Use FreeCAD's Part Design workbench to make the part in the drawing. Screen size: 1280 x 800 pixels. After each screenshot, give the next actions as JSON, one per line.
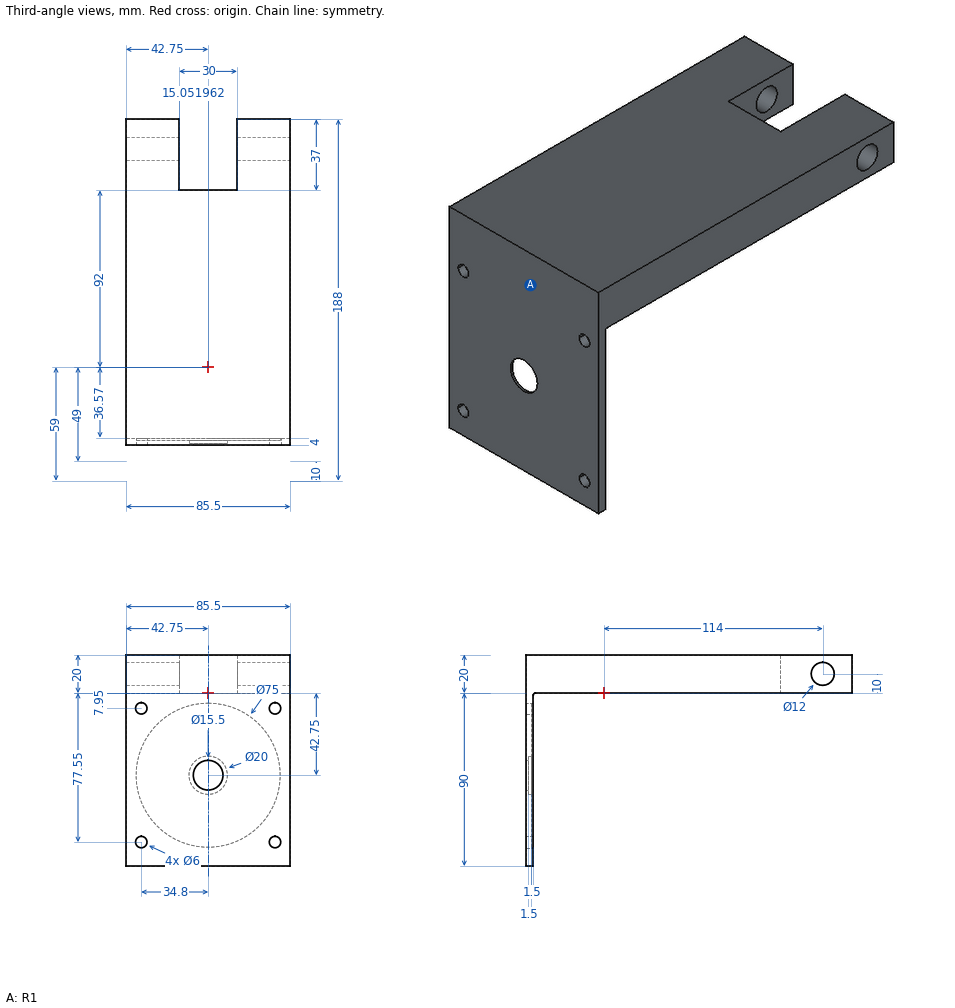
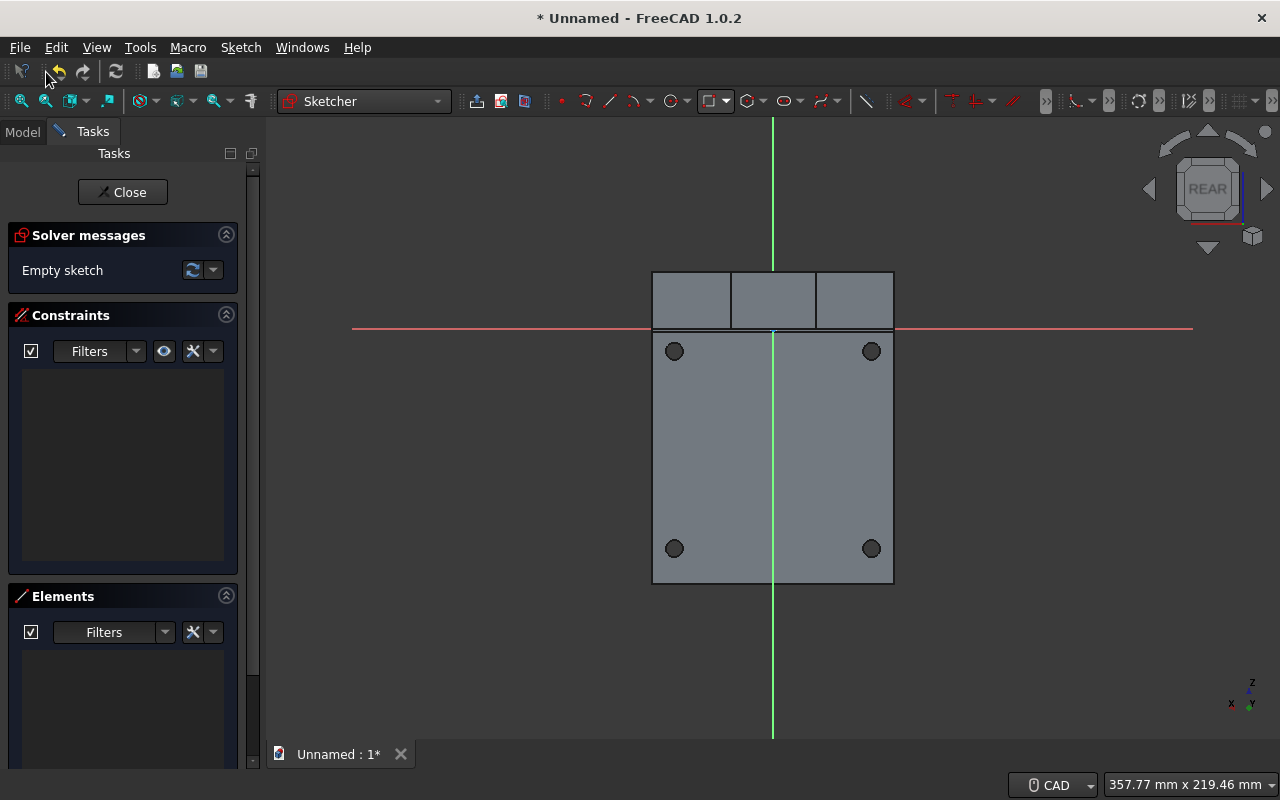
{"action": "scroll", "coordinate": [856, 460], "scroll_direction": "up", "scroll_amount": 3}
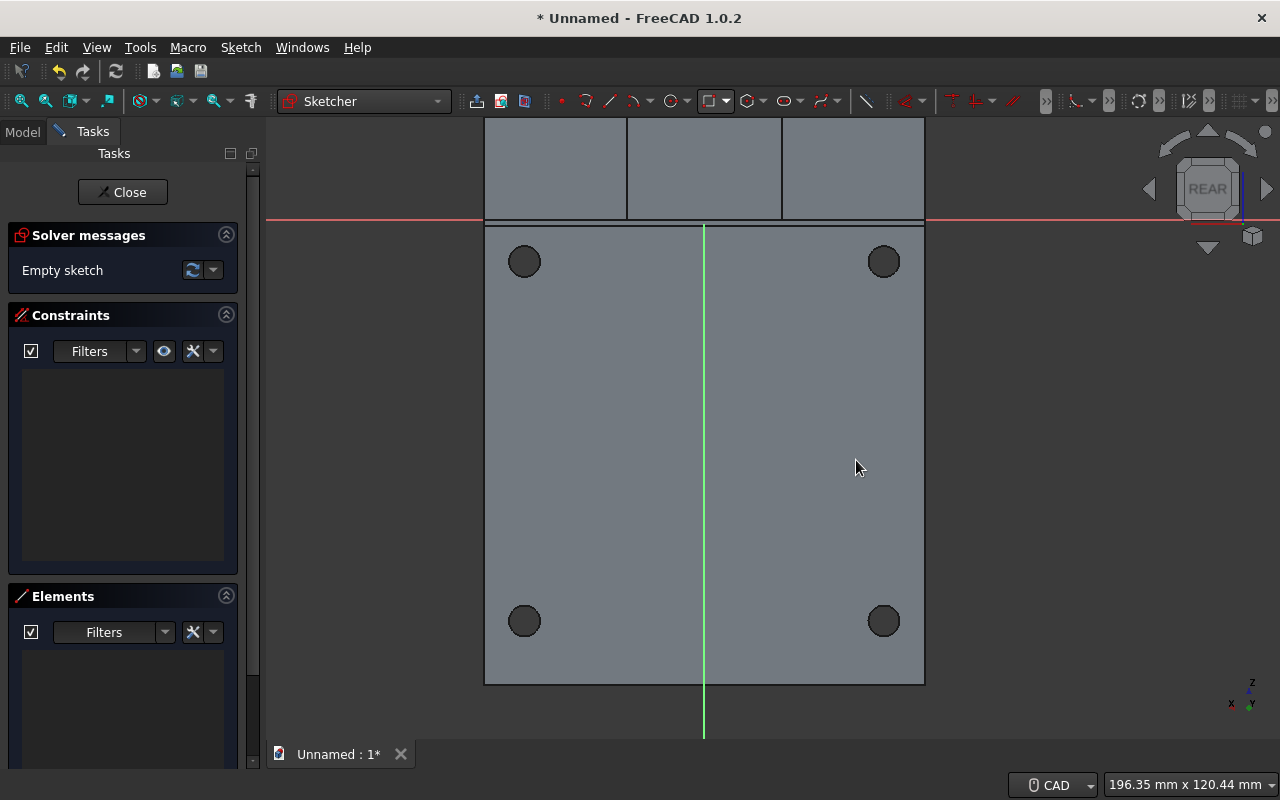
{"action": "key", "text": "g c"}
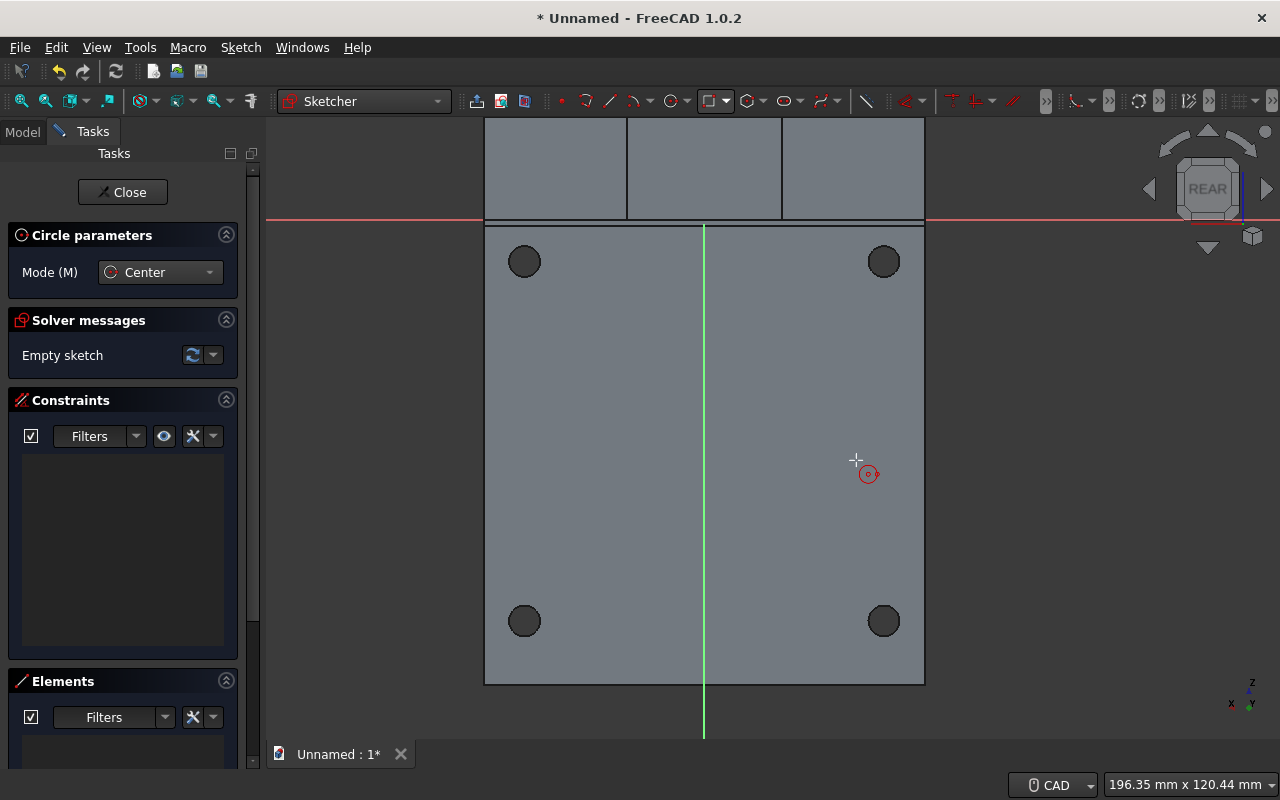
{"action": "left_click", "coordinate": [704, 441]}
{"action": "mouse_move", "coordinate": [841, 304]}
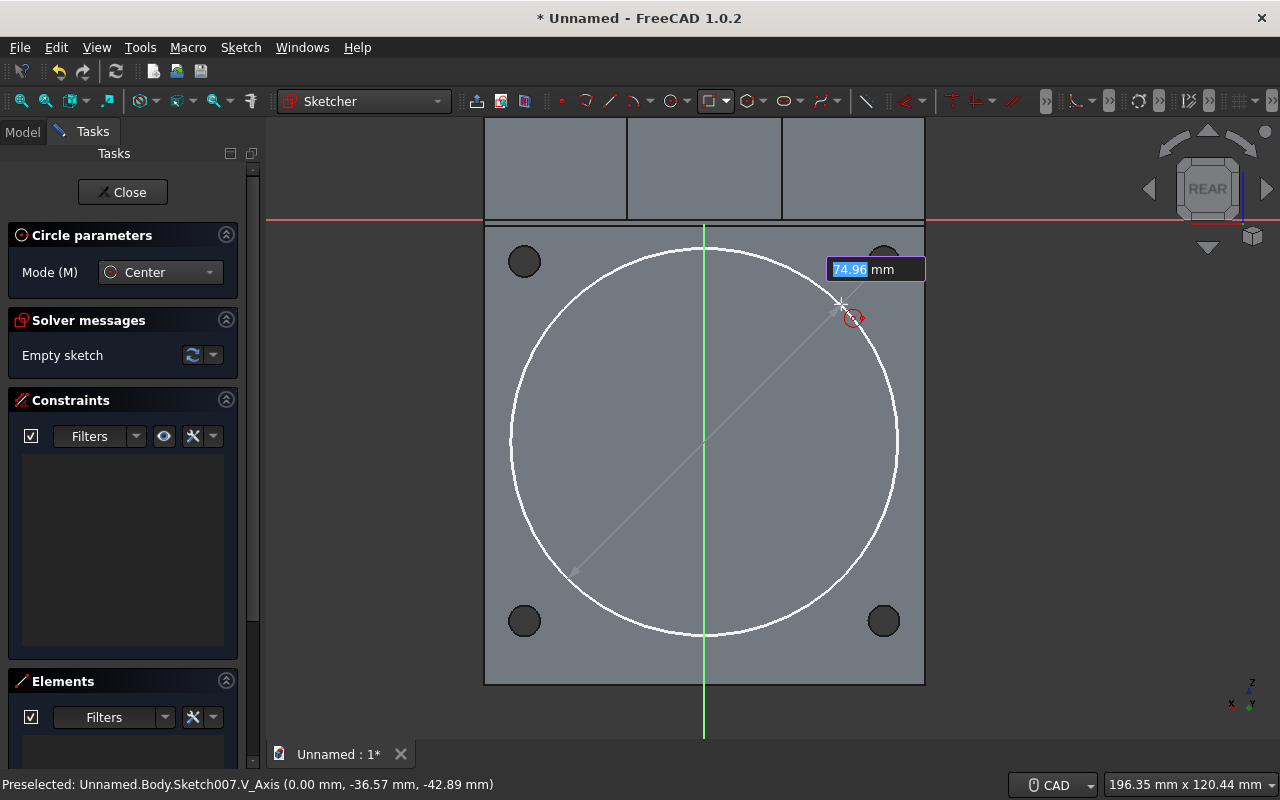
{"action": "type", "text": "75"}
{"action": "key", "text": "Return"}
{"action": "key", "text": "Escape"}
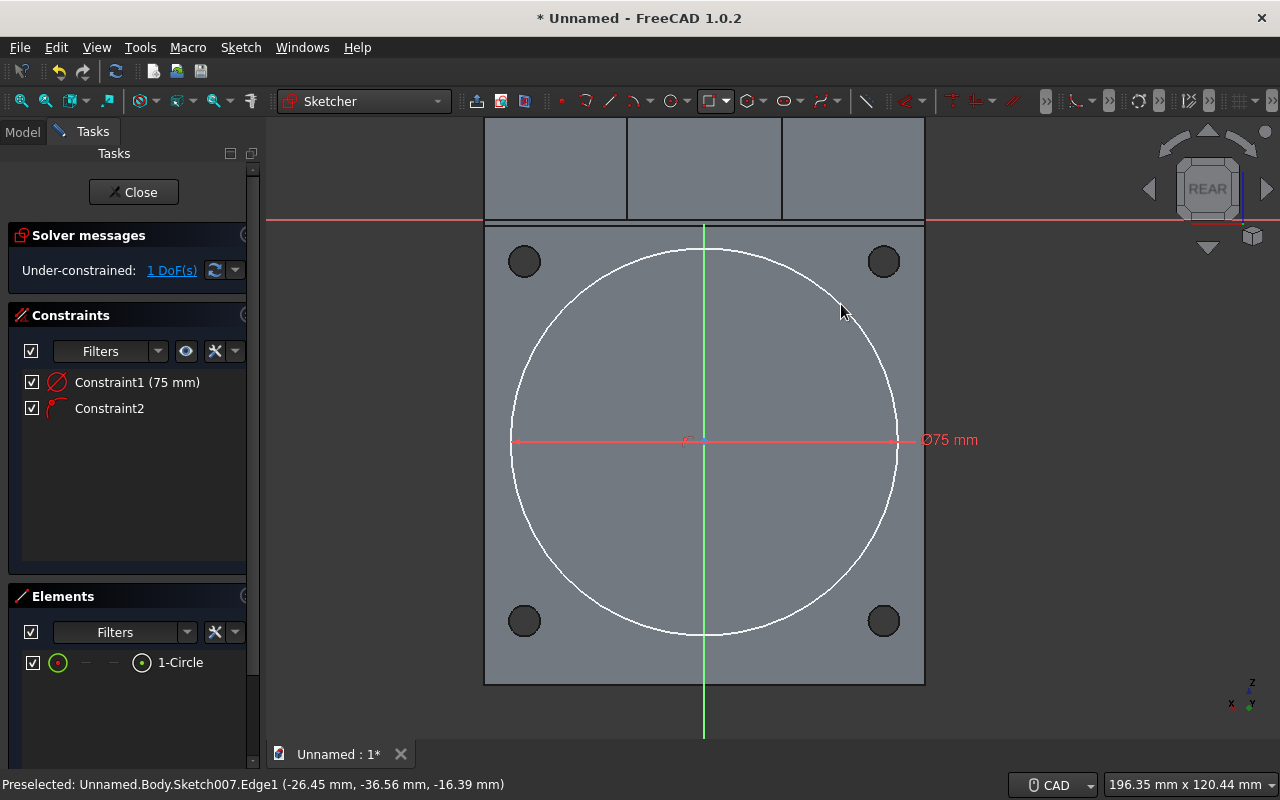
{"action": "key", "text": "d"}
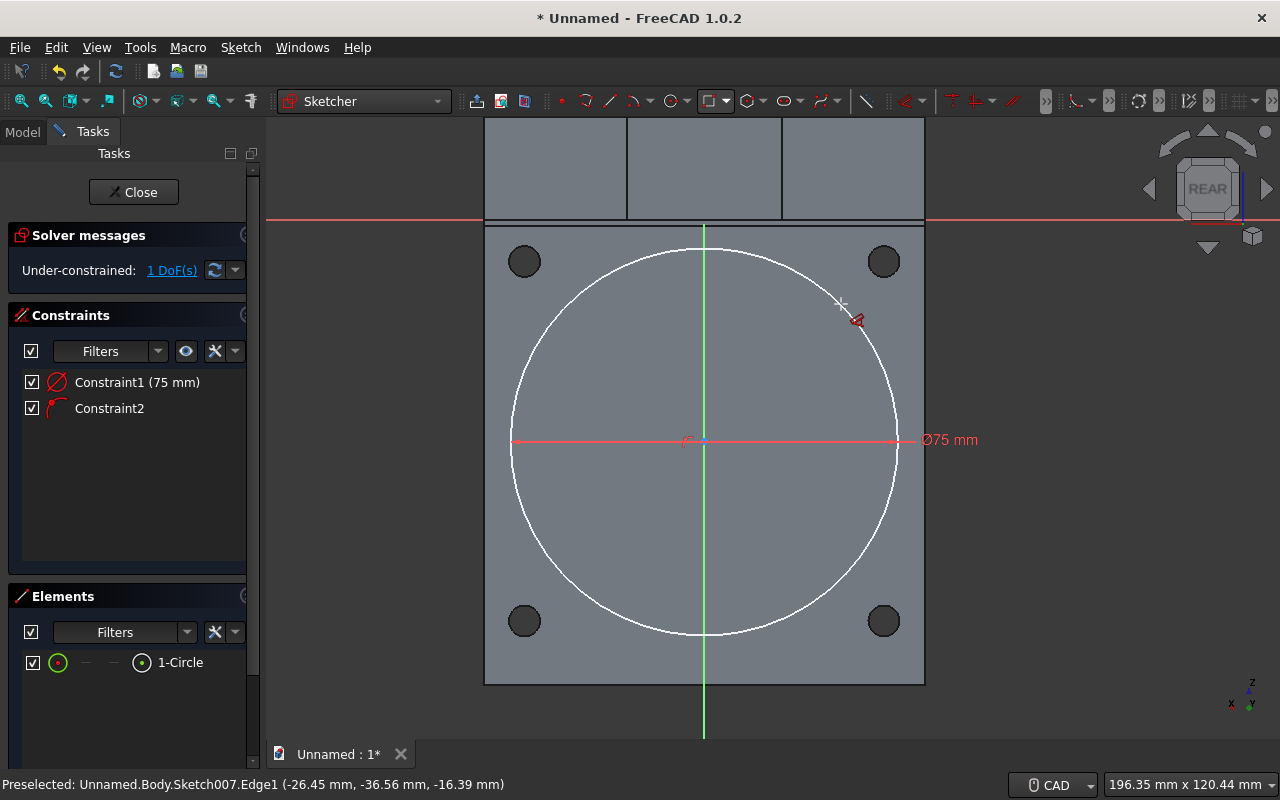
{"action": "left_click", "coordinate": [704, 442]}
{"action": "left_click", "coordinate": [738, 331]}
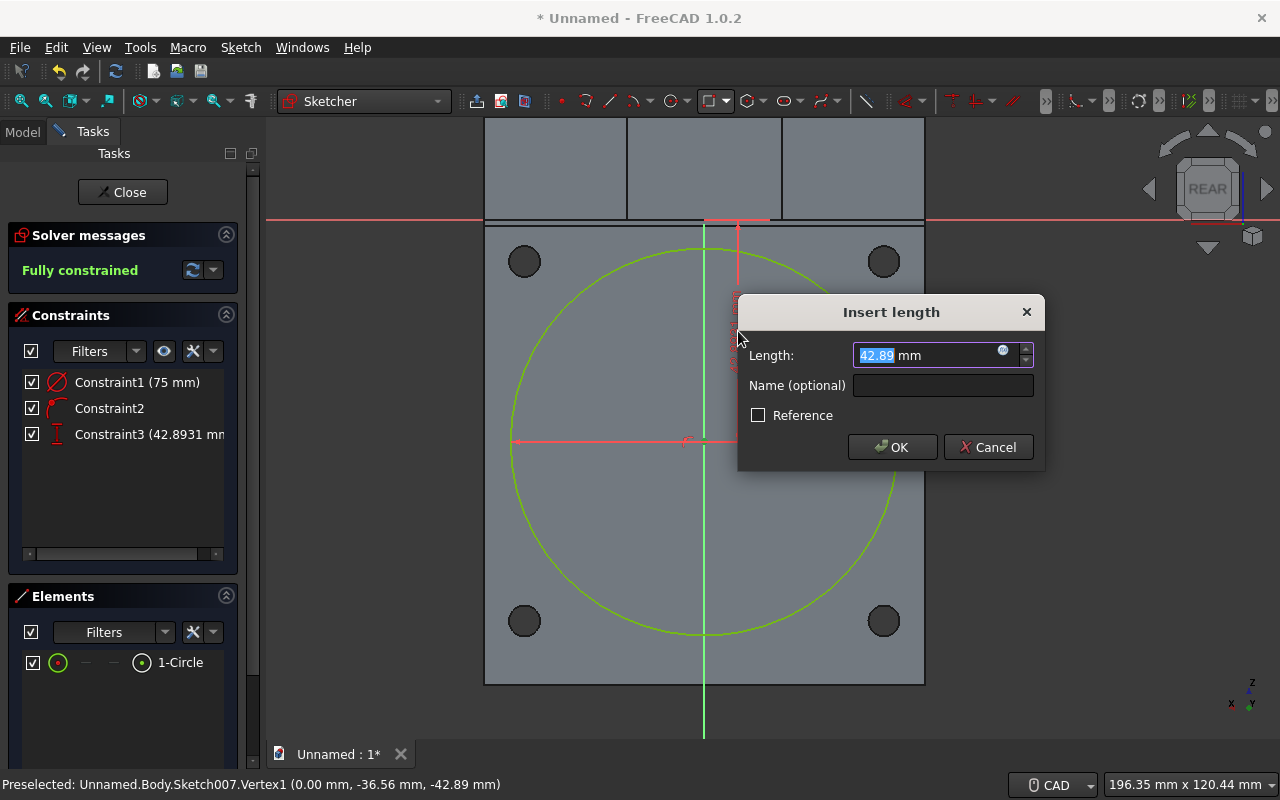
{"action": "type", "text": "42.75"}
{"action": "key", "text": "Return"}
{"action": "key", "text": "Escape"}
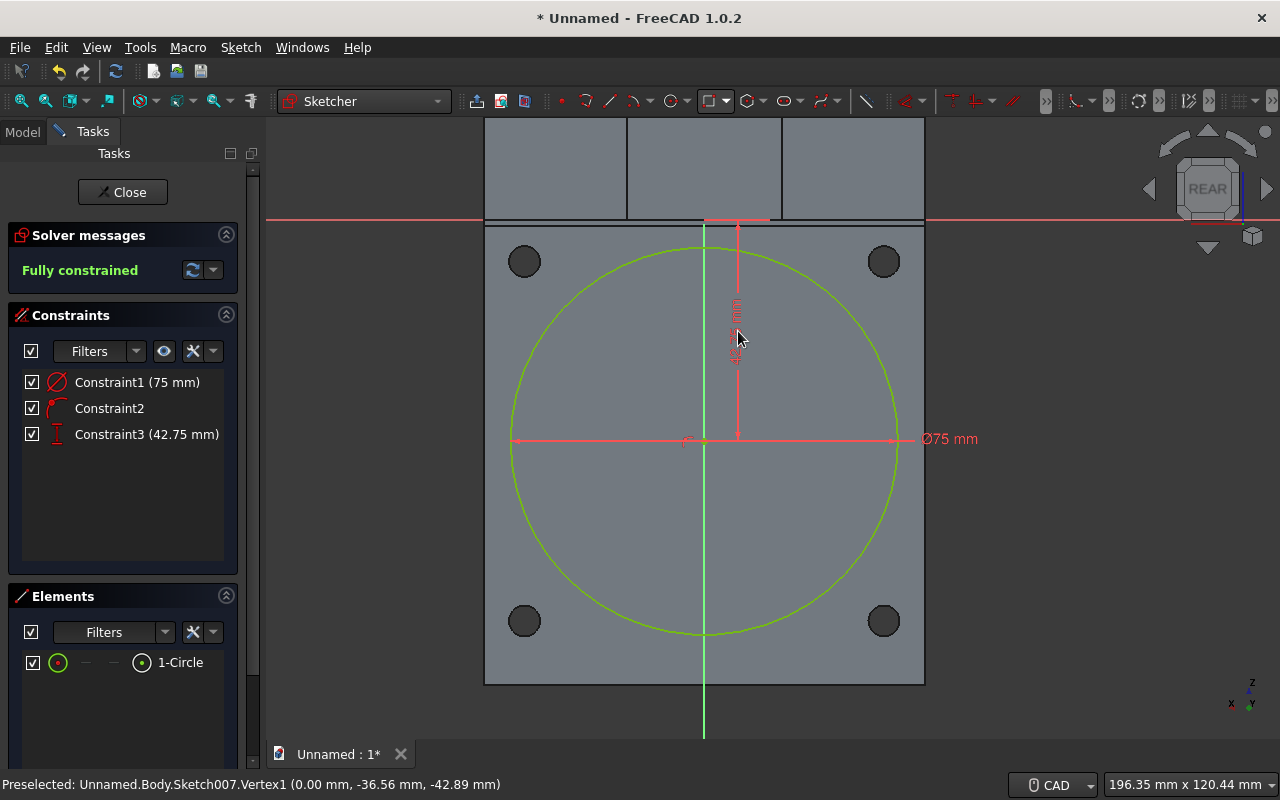
{"action": "left_click", "coordinate": [123, 192]}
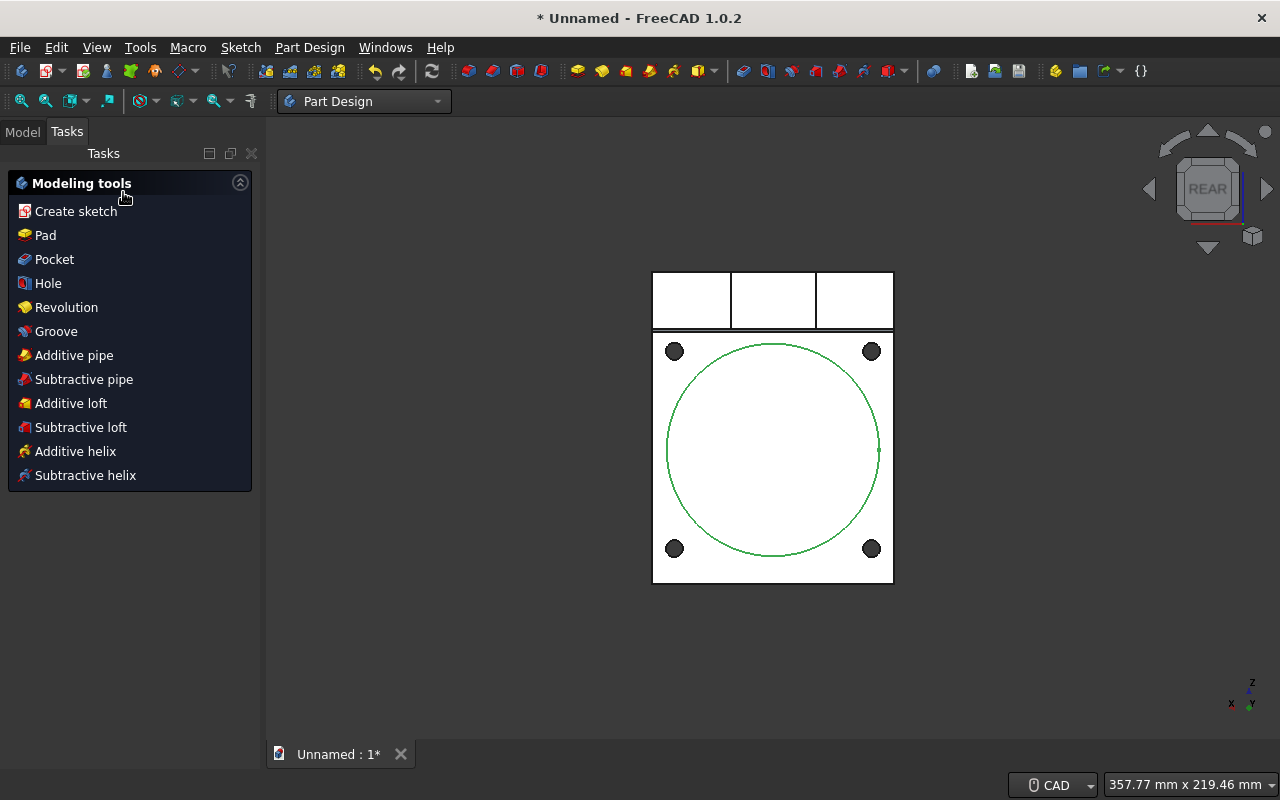
{"action": "left_click", "coordinate": [744, 72]}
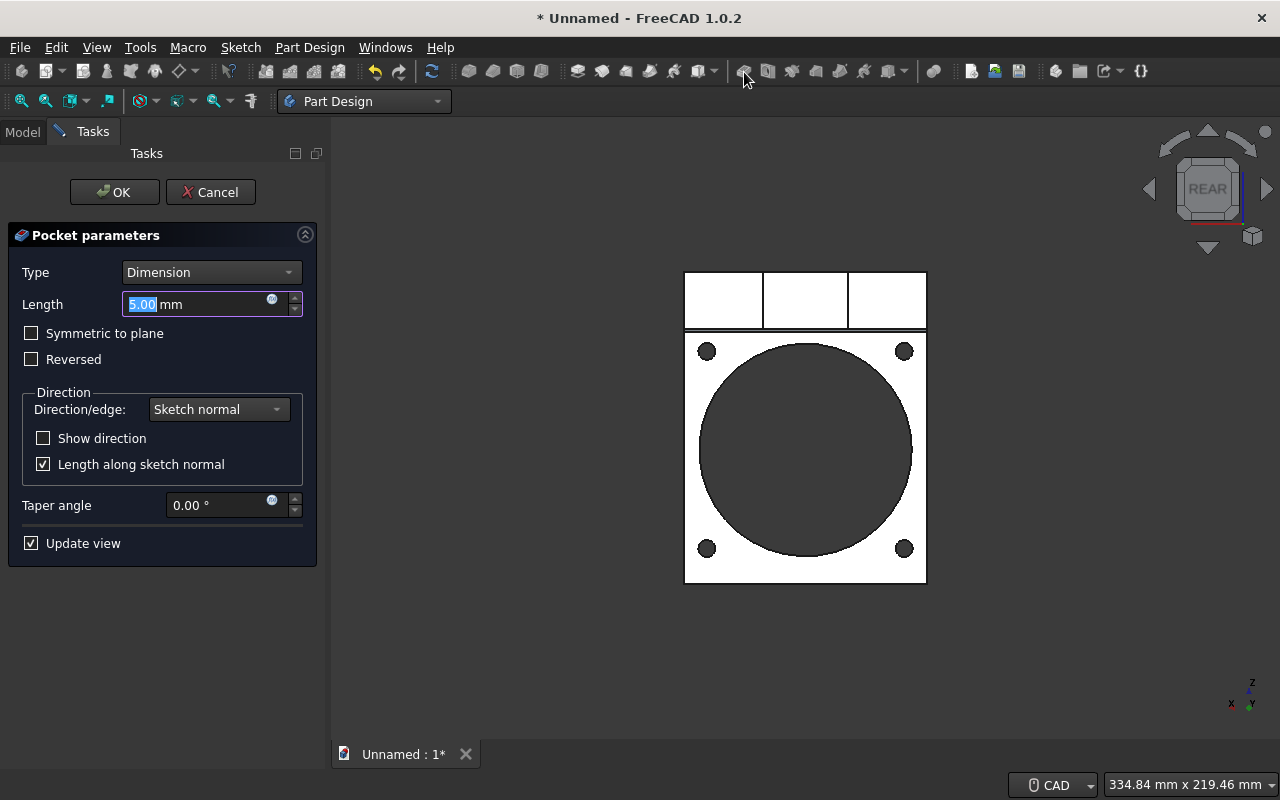
{"action": "type", "text": "1.5"}
{"action": "key", "text": "Tab"}